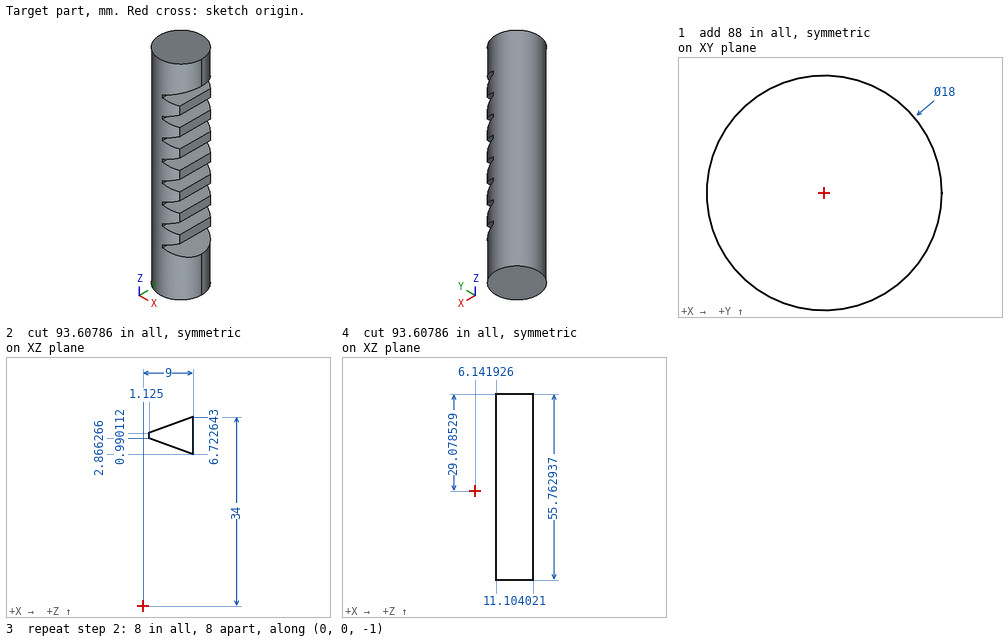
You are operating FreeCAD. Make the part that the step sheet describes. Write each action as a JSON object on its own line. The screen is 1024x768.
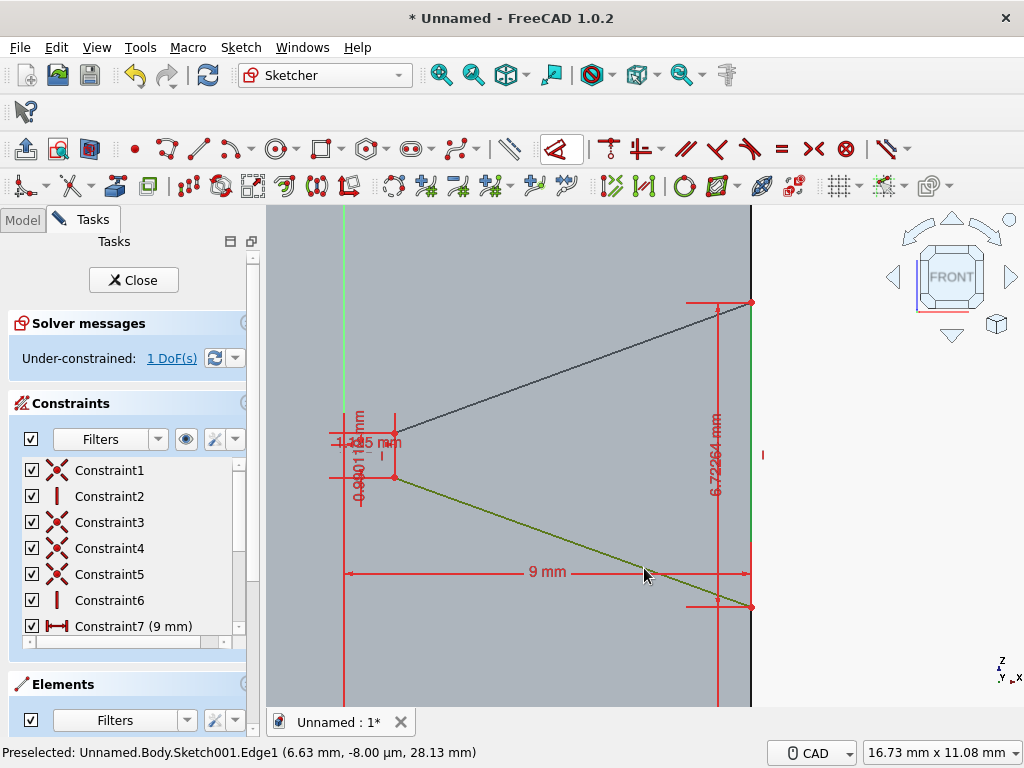
{"action": "key", "text": "i"}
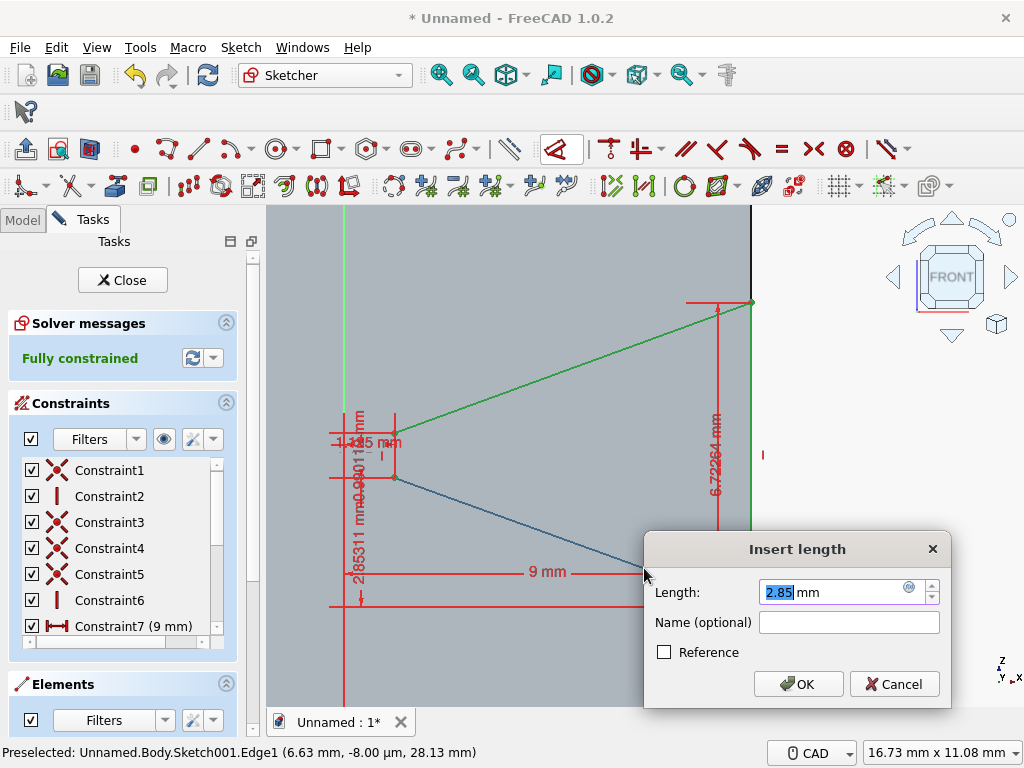
{"action": "type", "text": "2.866266"}
{"action": "key", "text": "Return"}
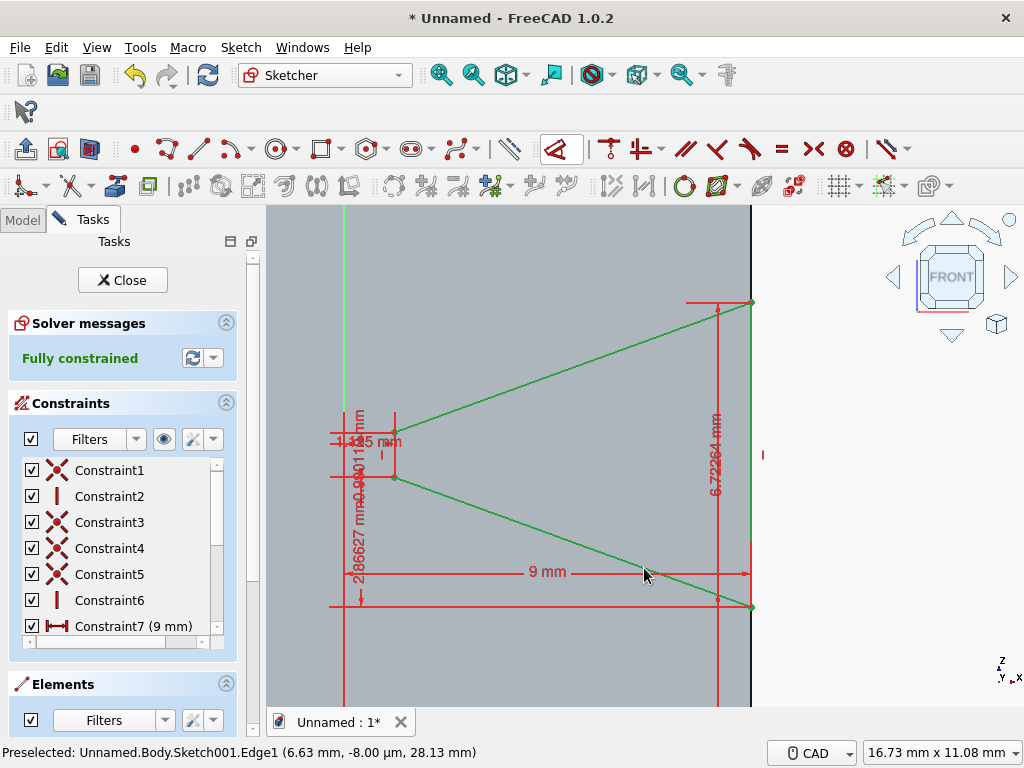
{"action": "left_click", "coordinate": [123, 280]}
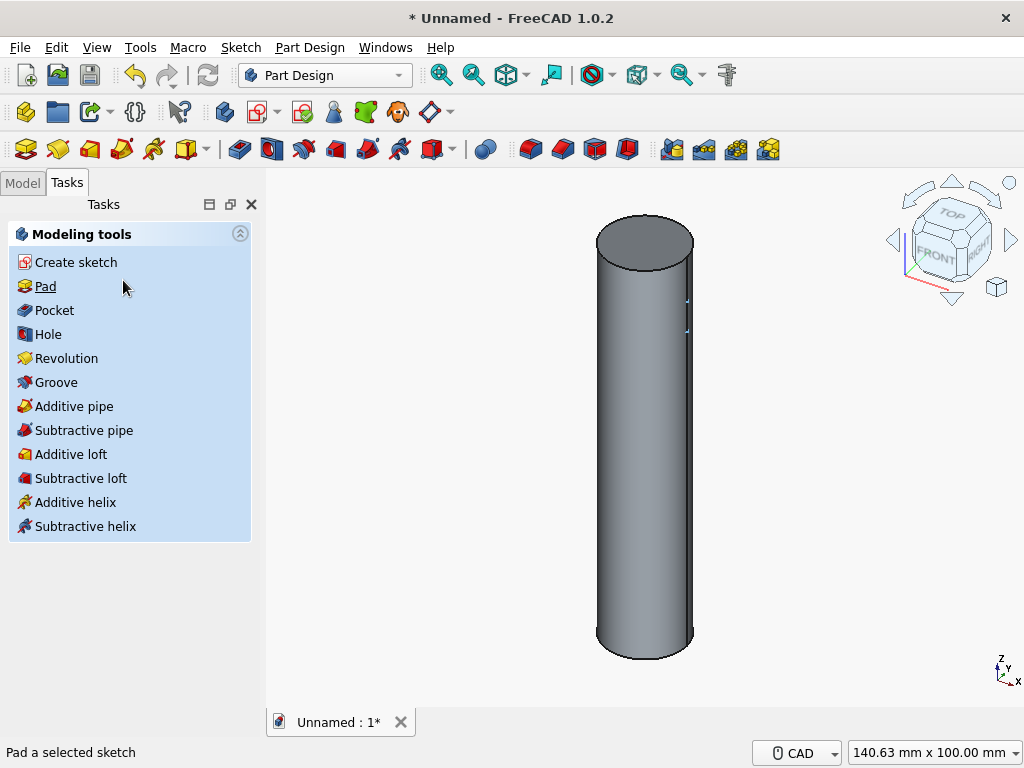
{"action": "left_click", "coordinate": [240, 150]}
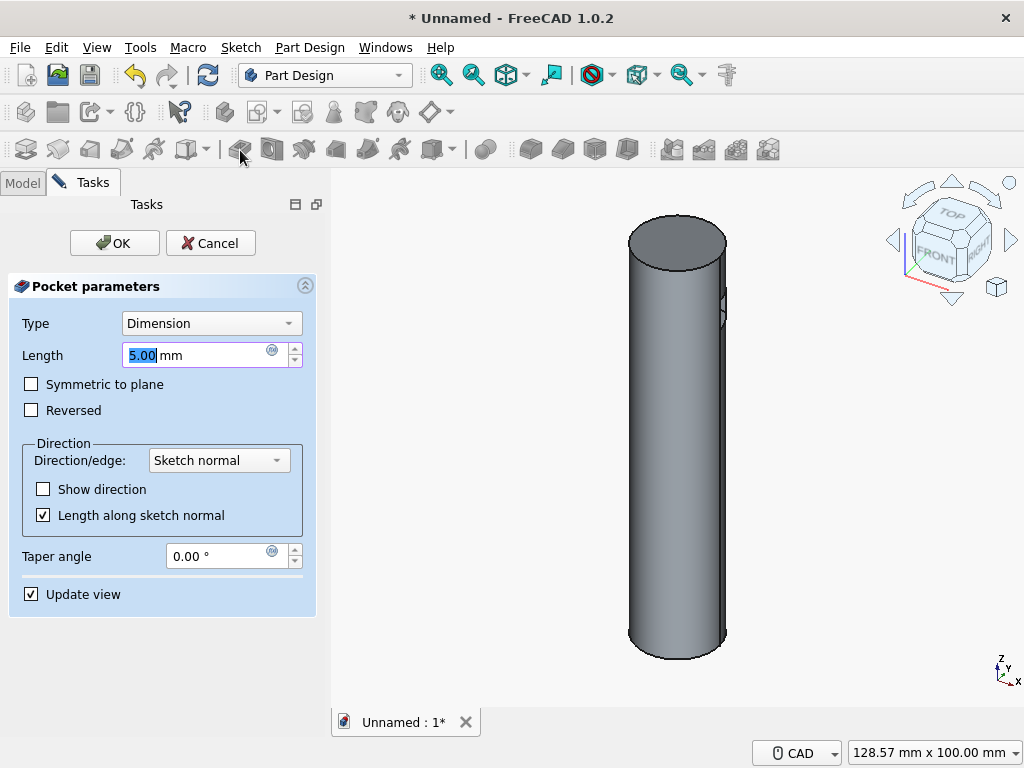
{"action": "type", "text": "93.60786"}
{"action": "key", "text": "Tab"}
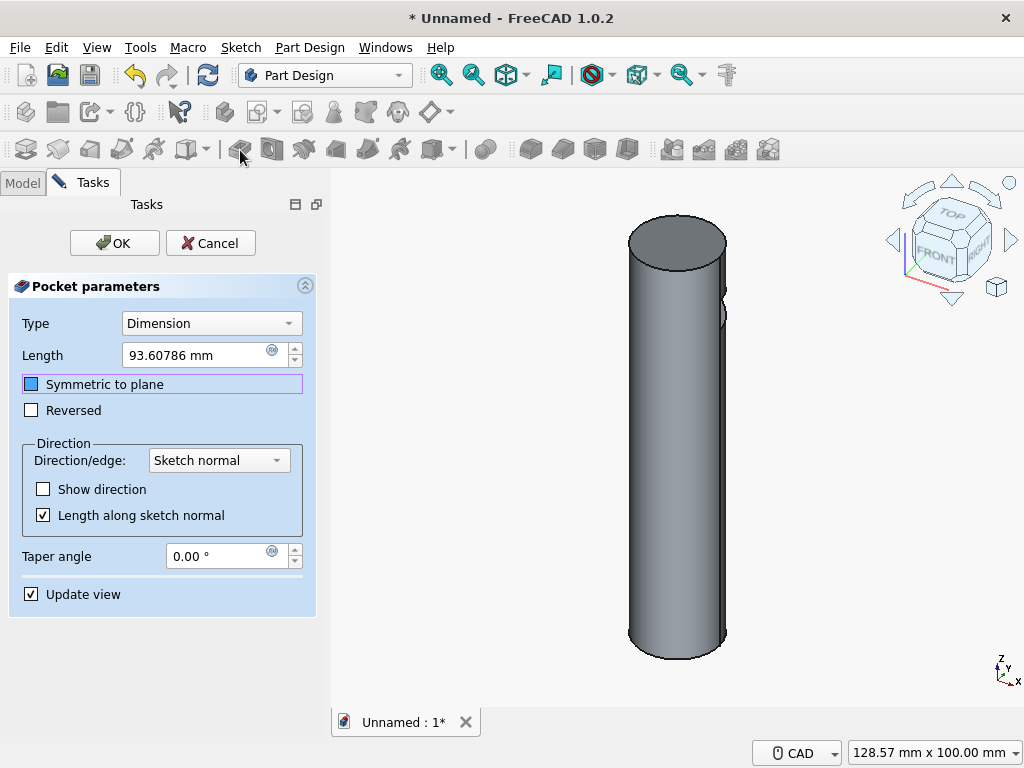
{"action": "left_click", "coordinate": [30, 384]}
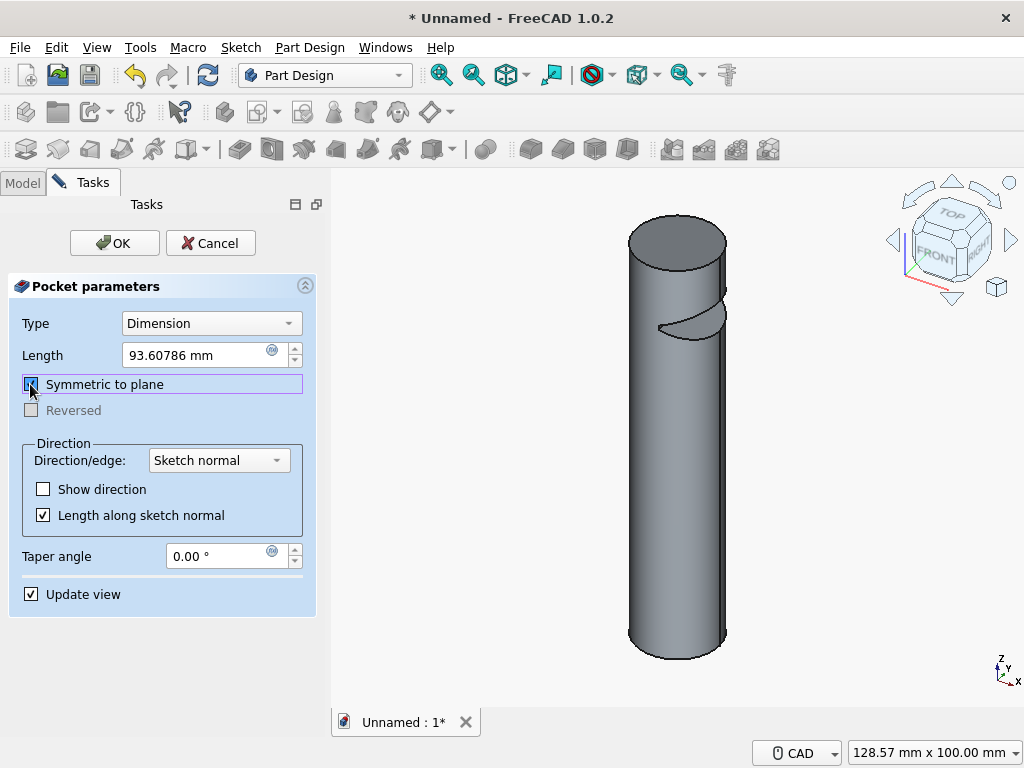
{"action": "left_click", "coordinate": [115, 243]}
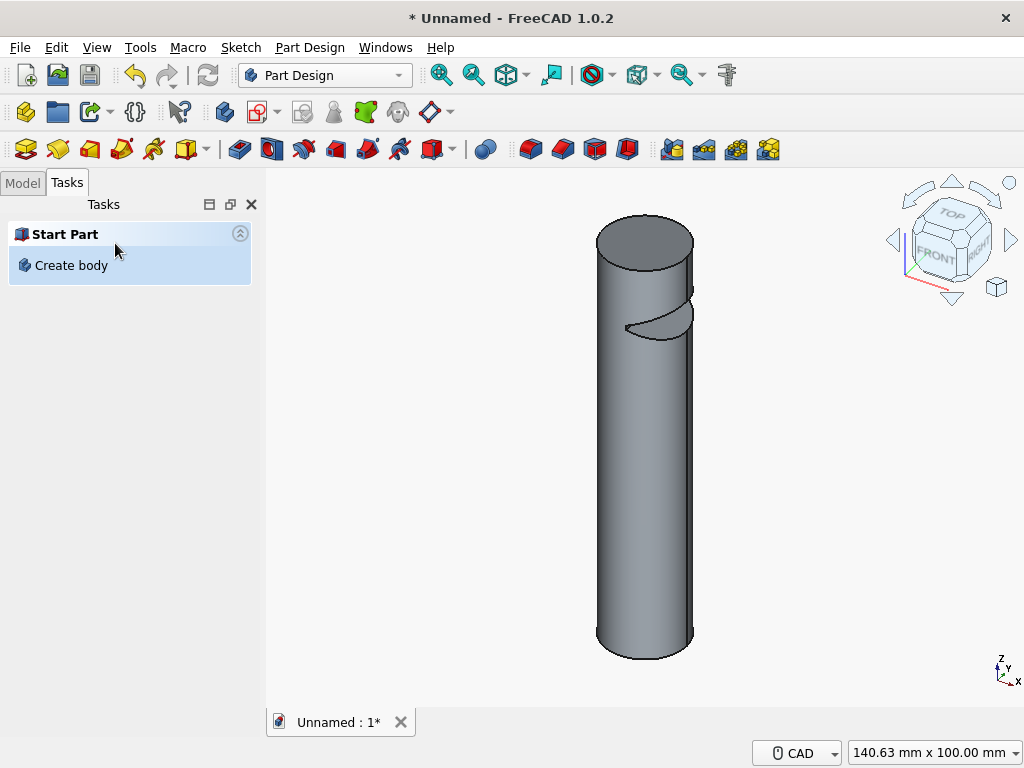
{"action": "left_click", "coordinate": [23, 182]}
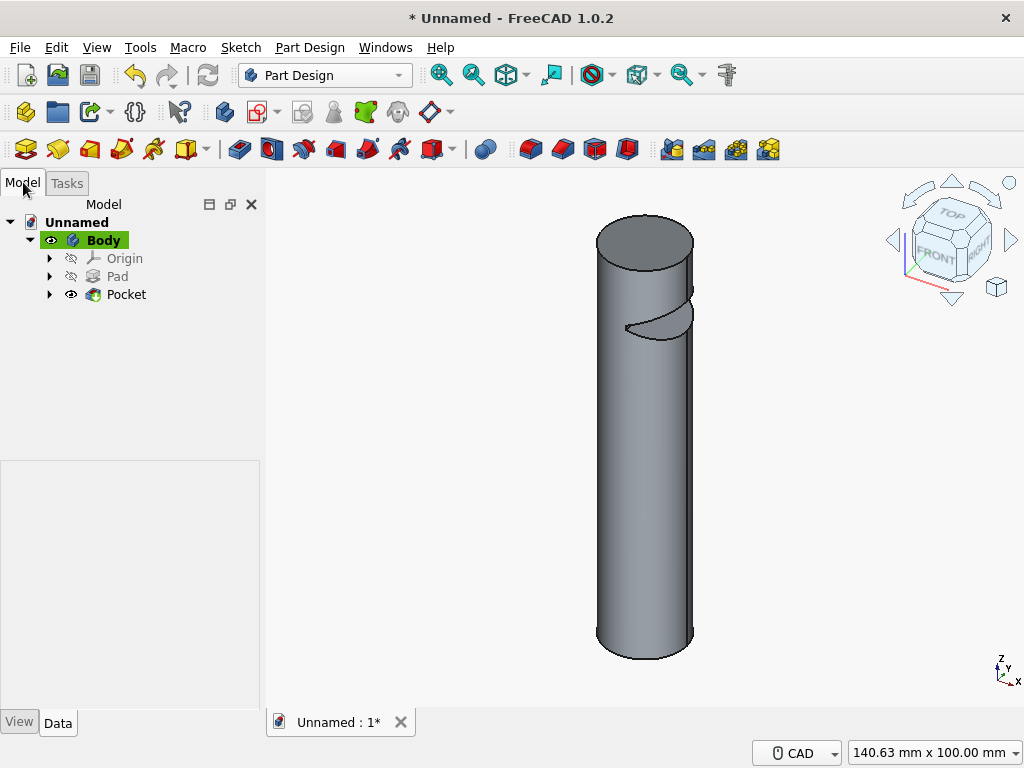
{"action": "left_click", "coordinate": [116, 294]}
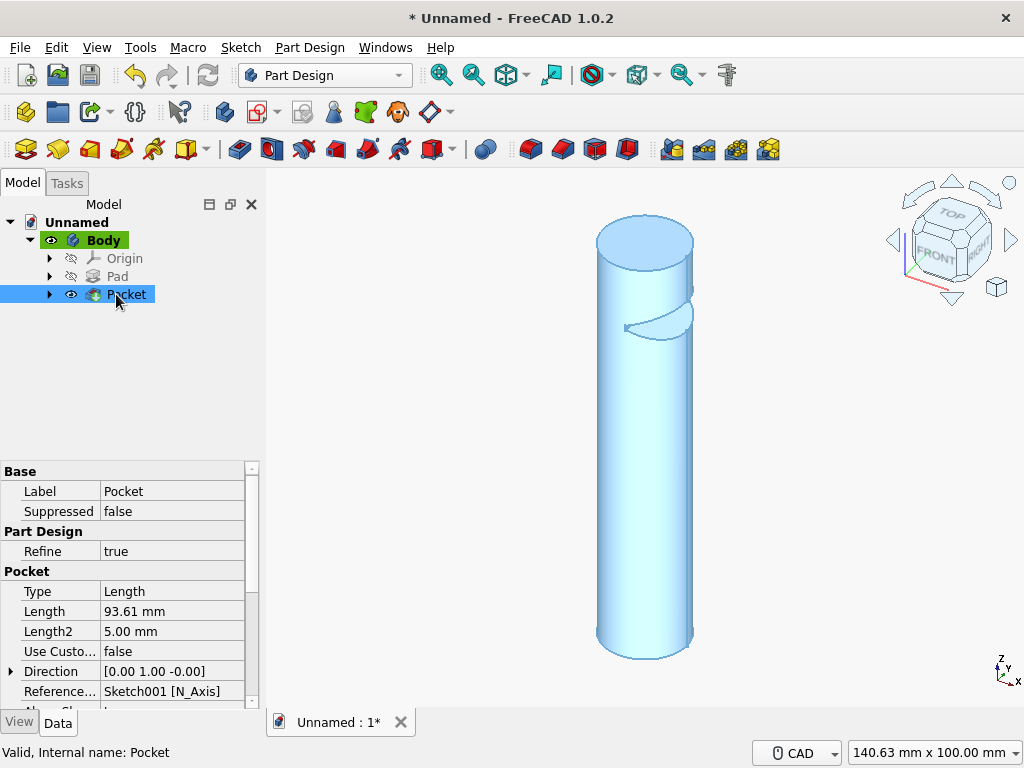
{"action": "left_click", "coordinate": [704, 150]}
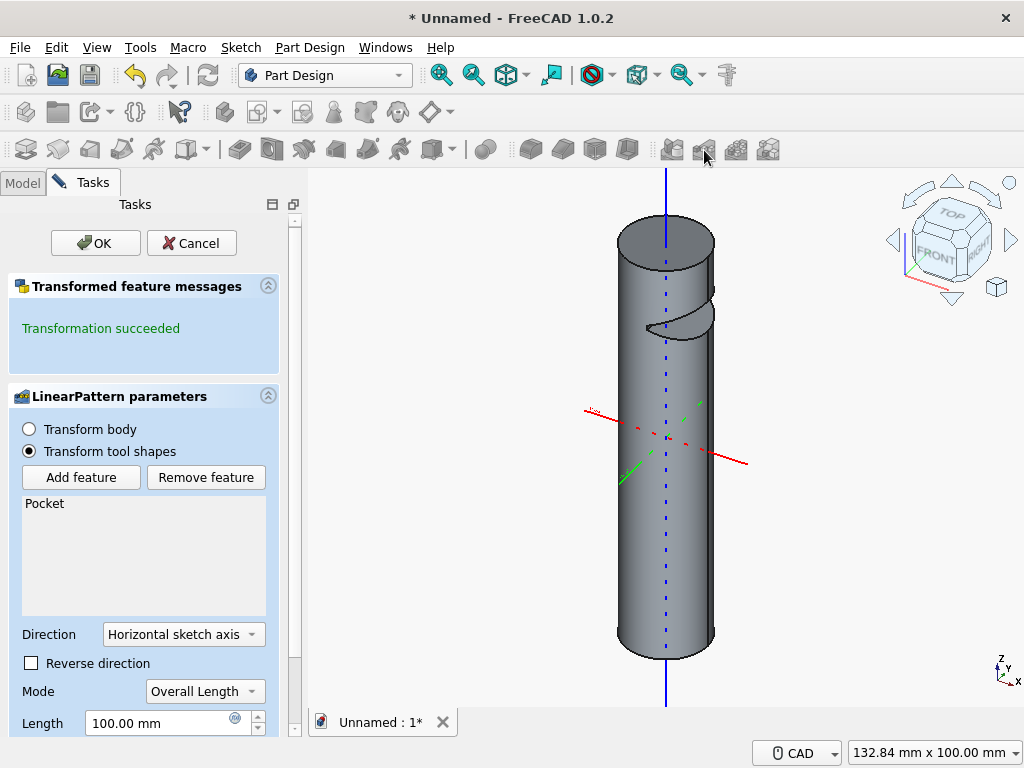
{"action": "left_click", "coordinate": [184, 634]}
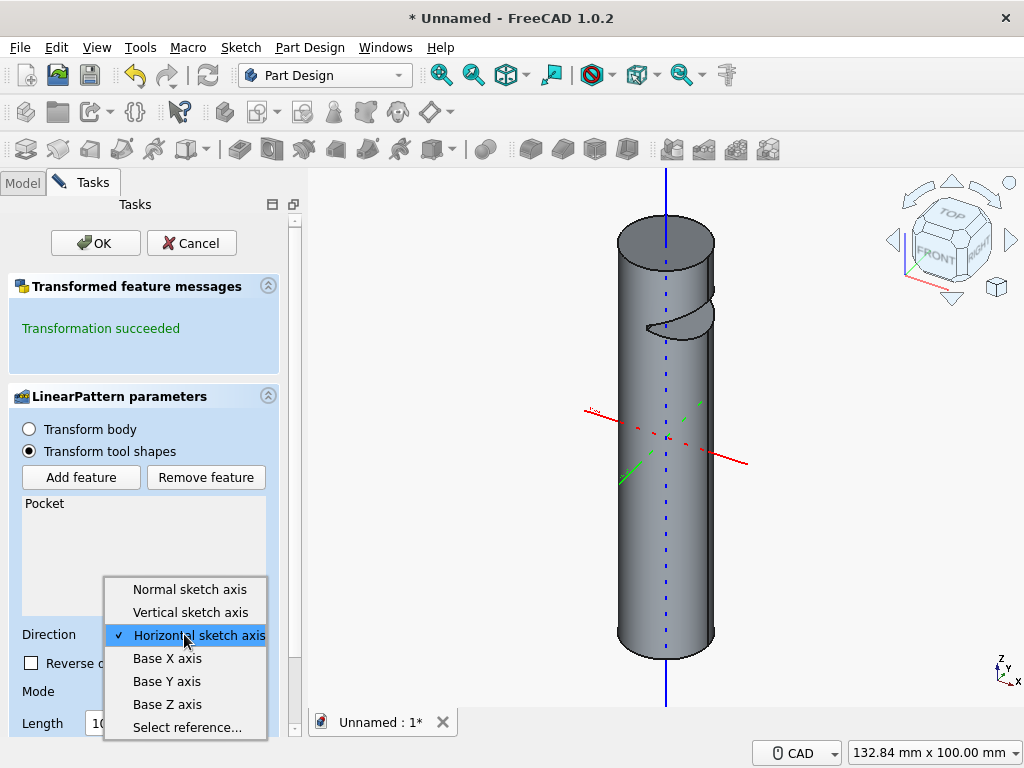
{"action": "left_click", "coordinate": [184, 704]}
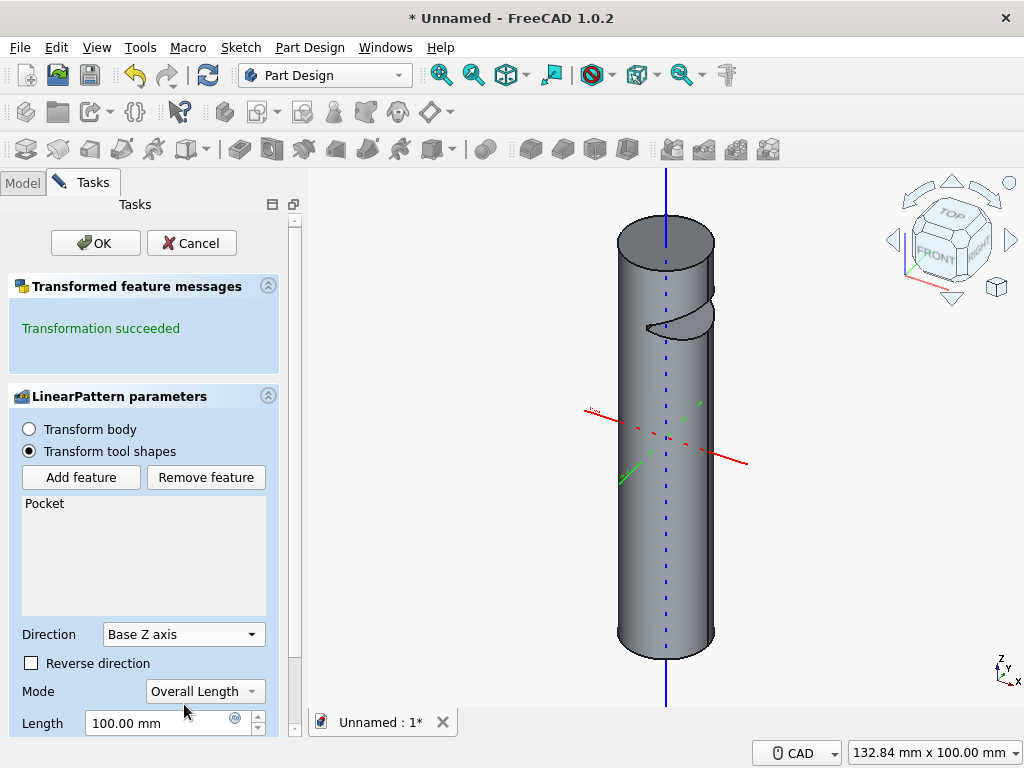
{"action": "left_click", "coordinate": [206, 692]}